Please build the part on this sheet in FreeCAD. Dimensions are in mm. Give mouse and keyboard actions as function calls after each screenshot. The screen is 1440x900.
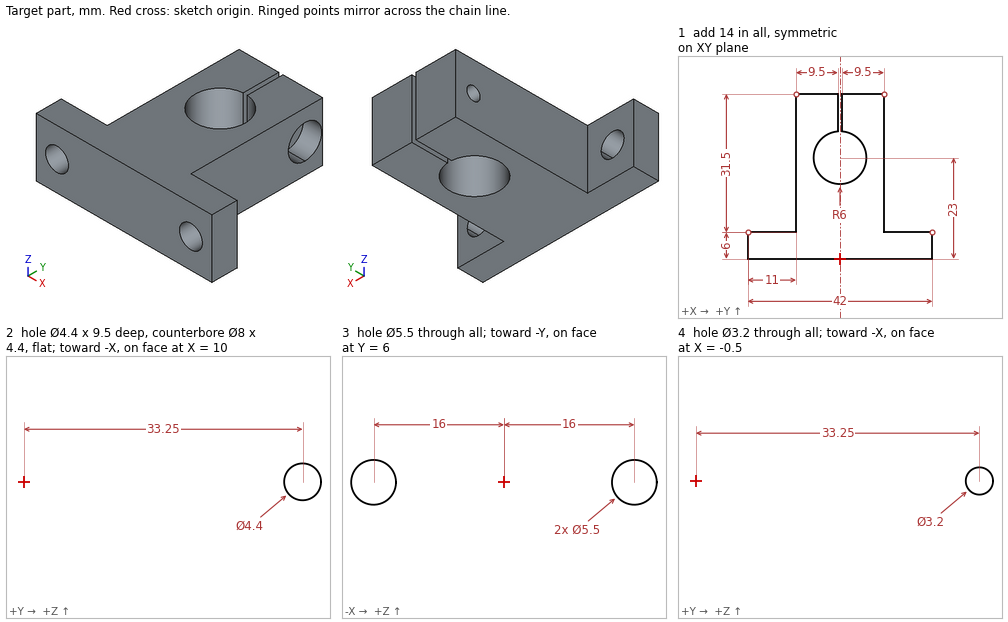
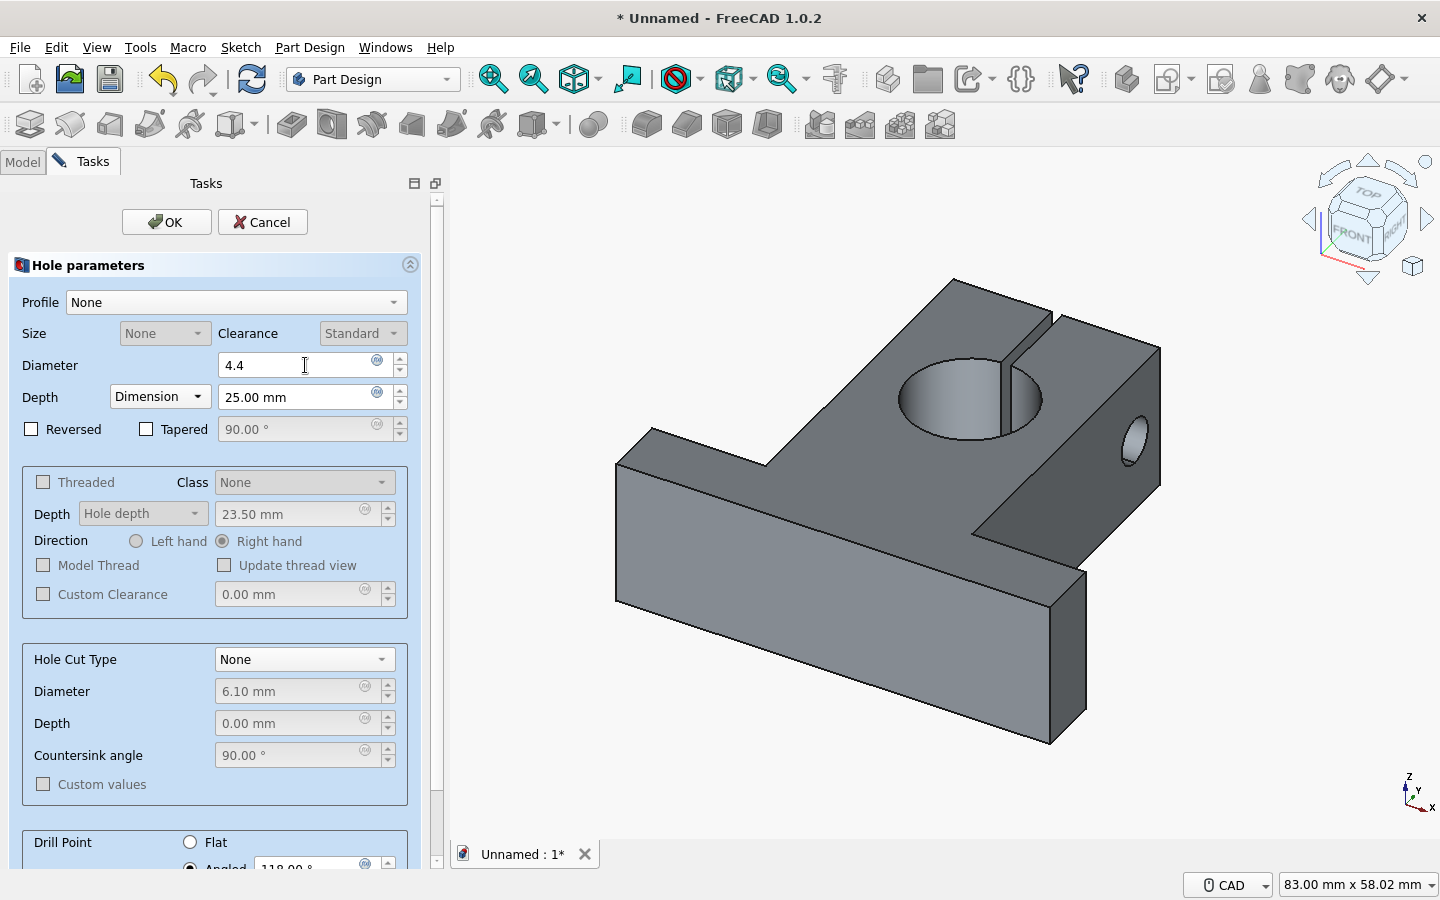
triple_click(305, 397)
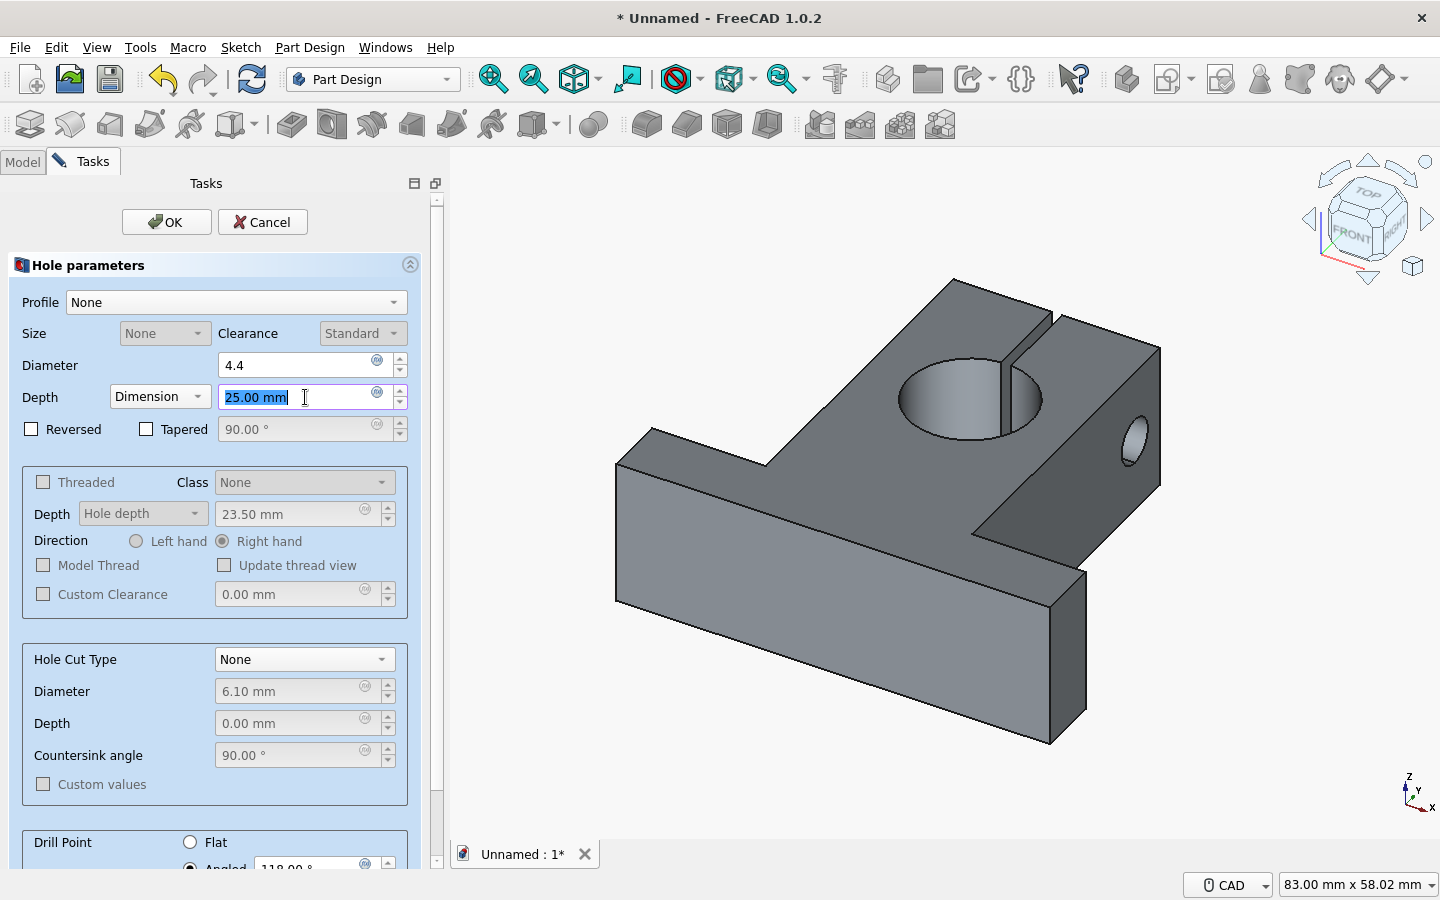
text(9.5)
key(Tab)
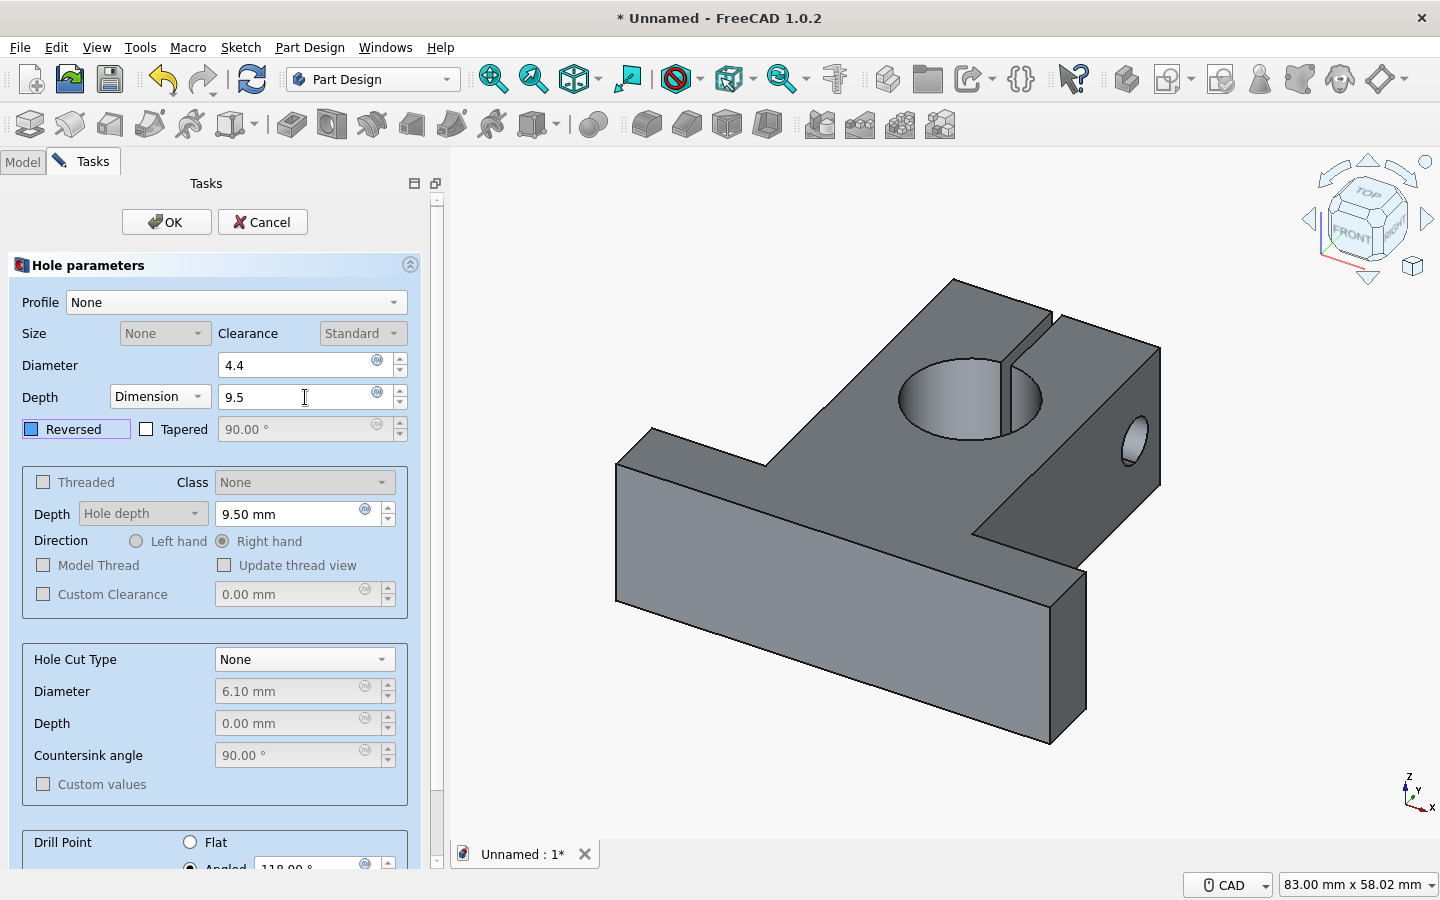
click(306, 660)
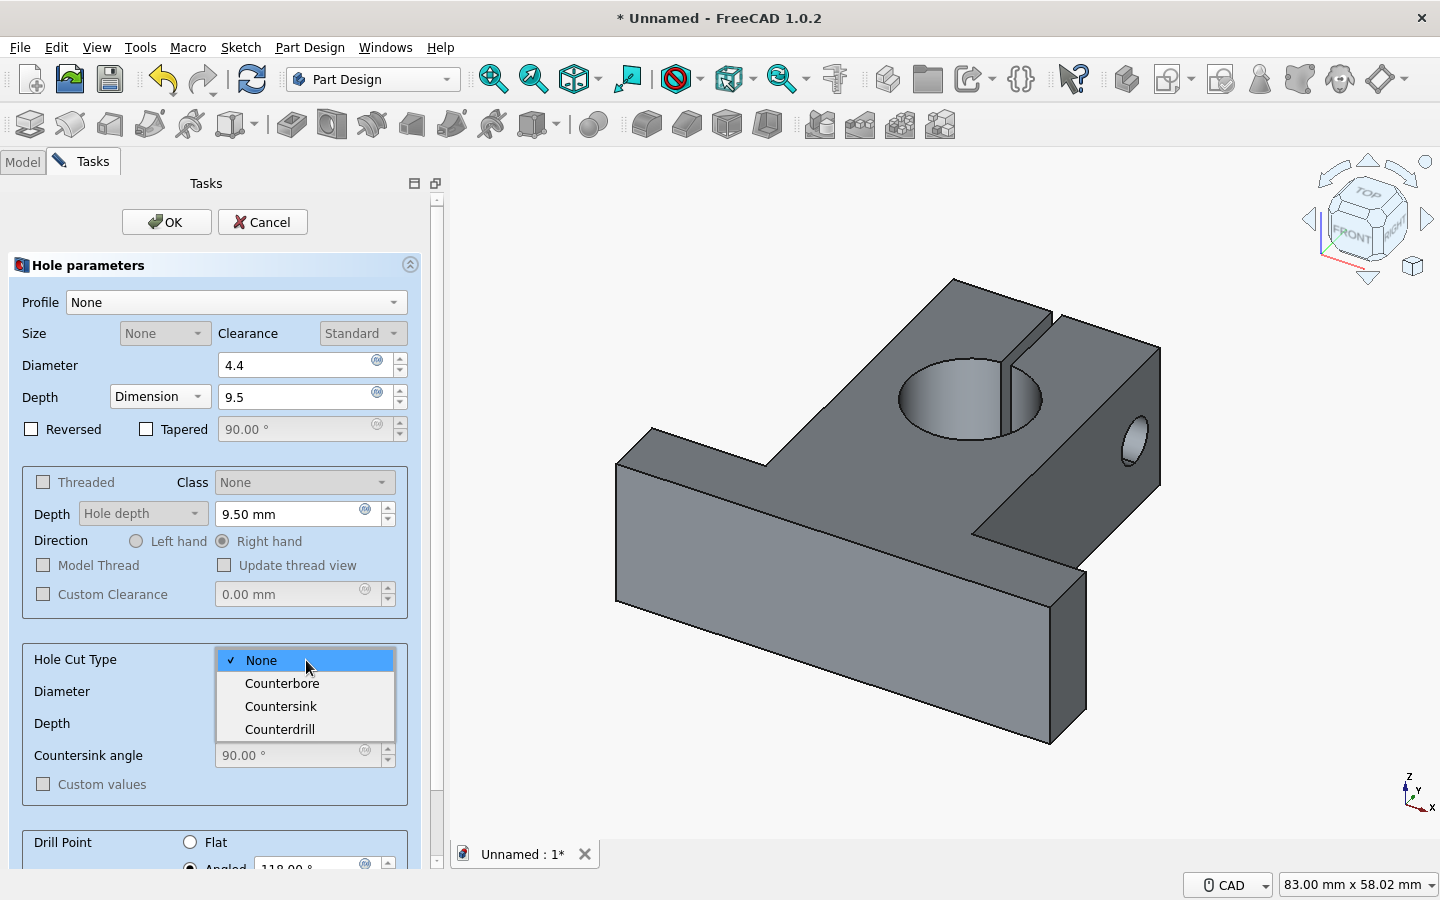
click(304, 684)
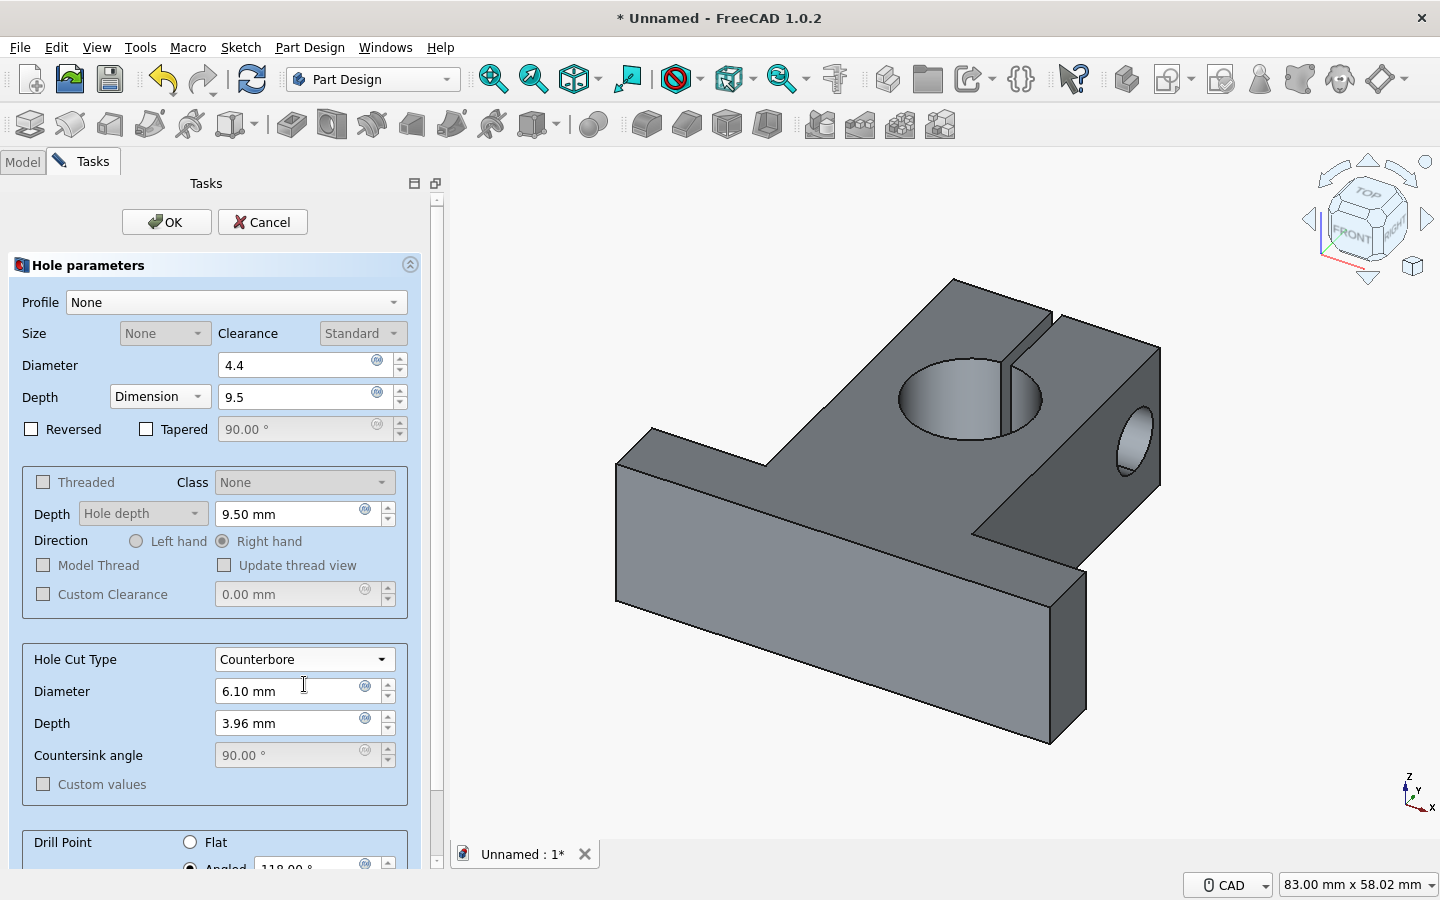
triple_click(298, 691)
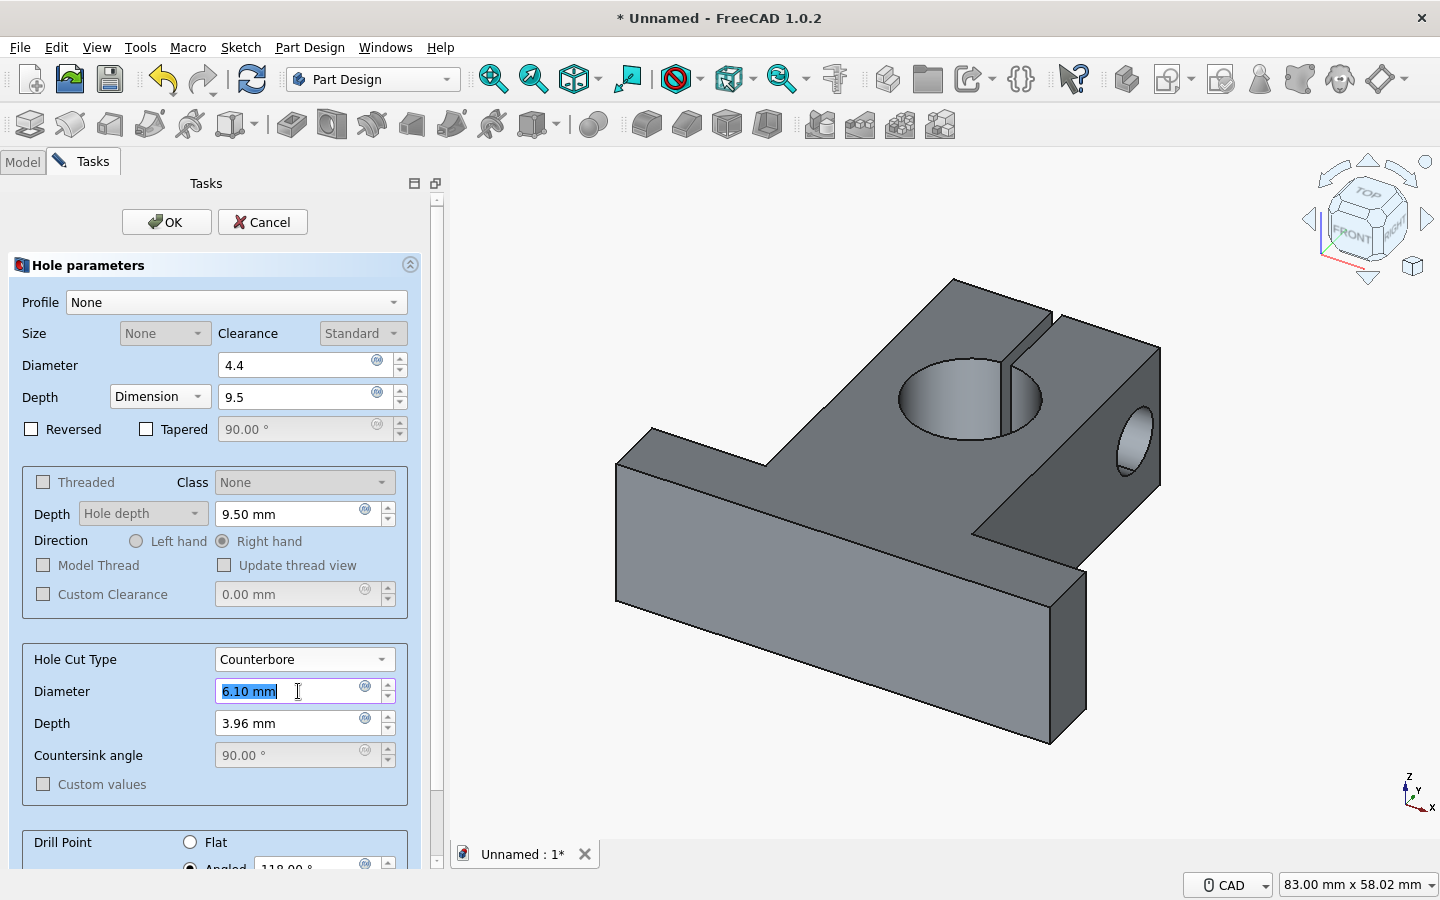
text(8)
key(Tab)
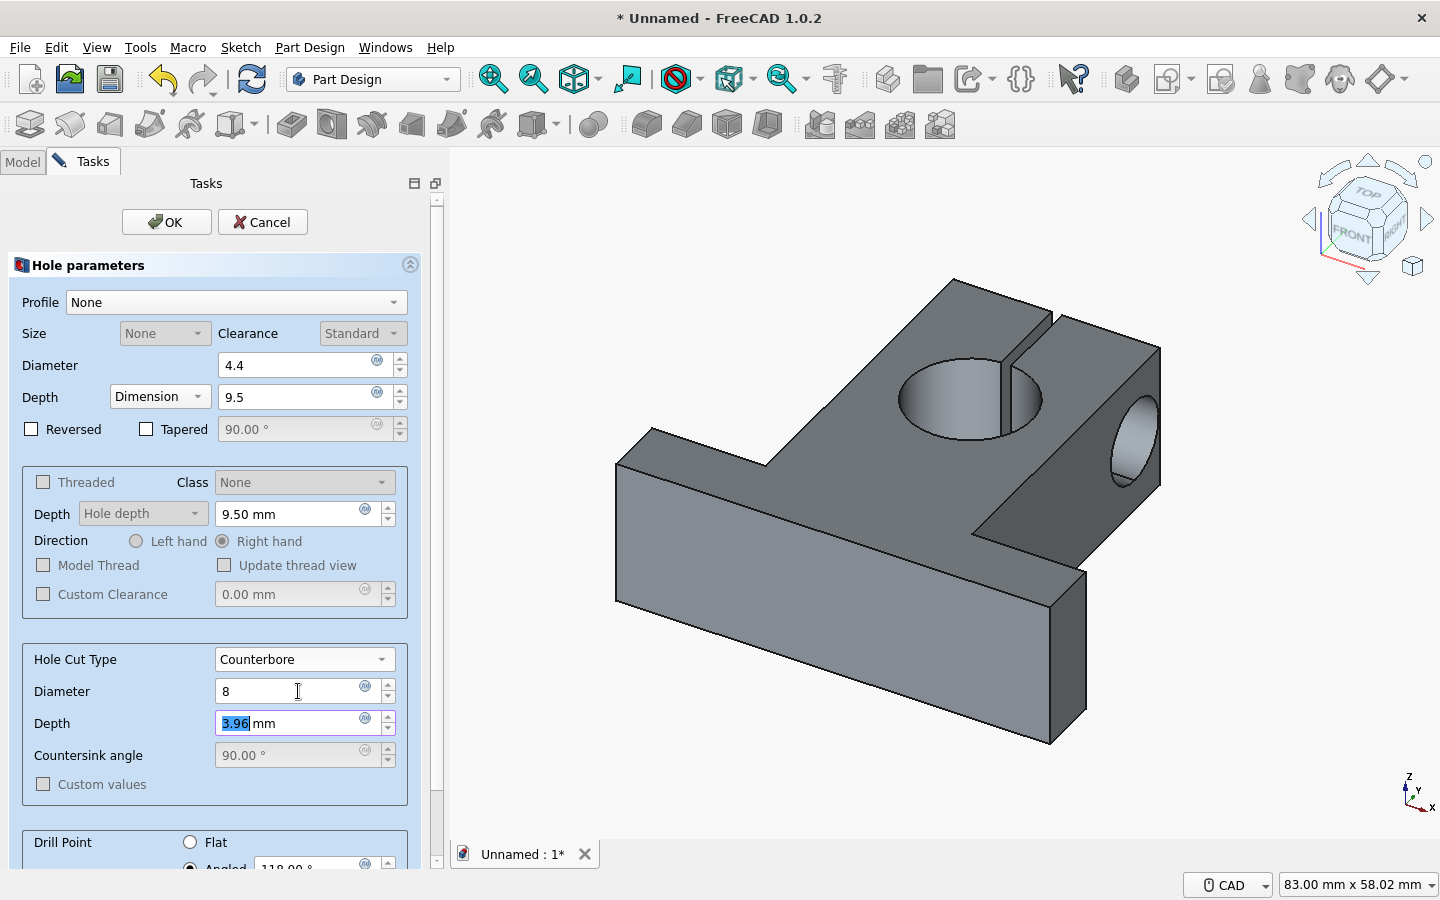
text(4.4)
key(Tab)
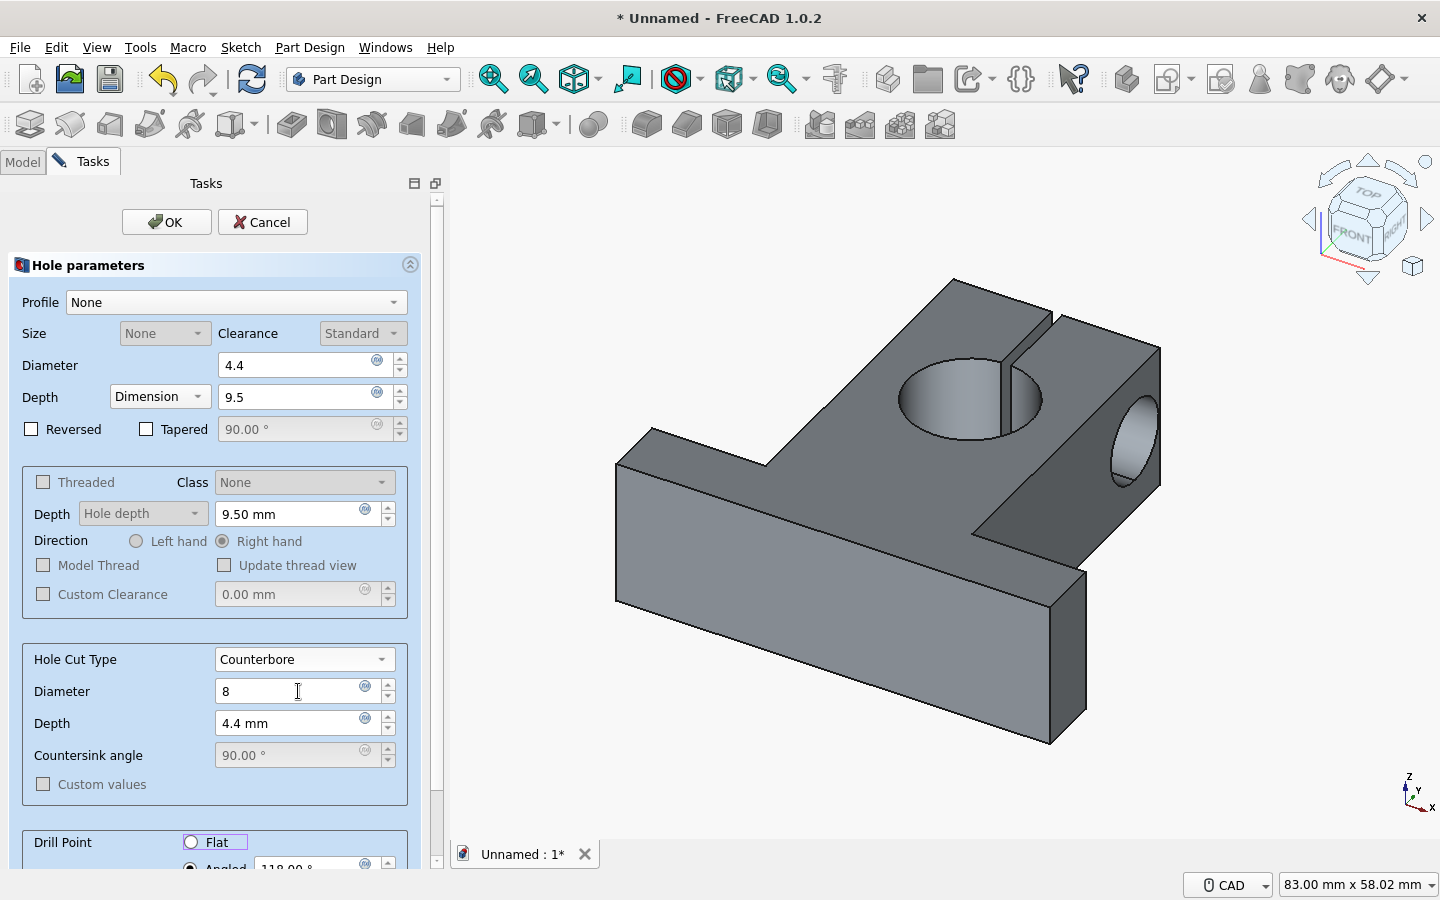
click(191, 842)